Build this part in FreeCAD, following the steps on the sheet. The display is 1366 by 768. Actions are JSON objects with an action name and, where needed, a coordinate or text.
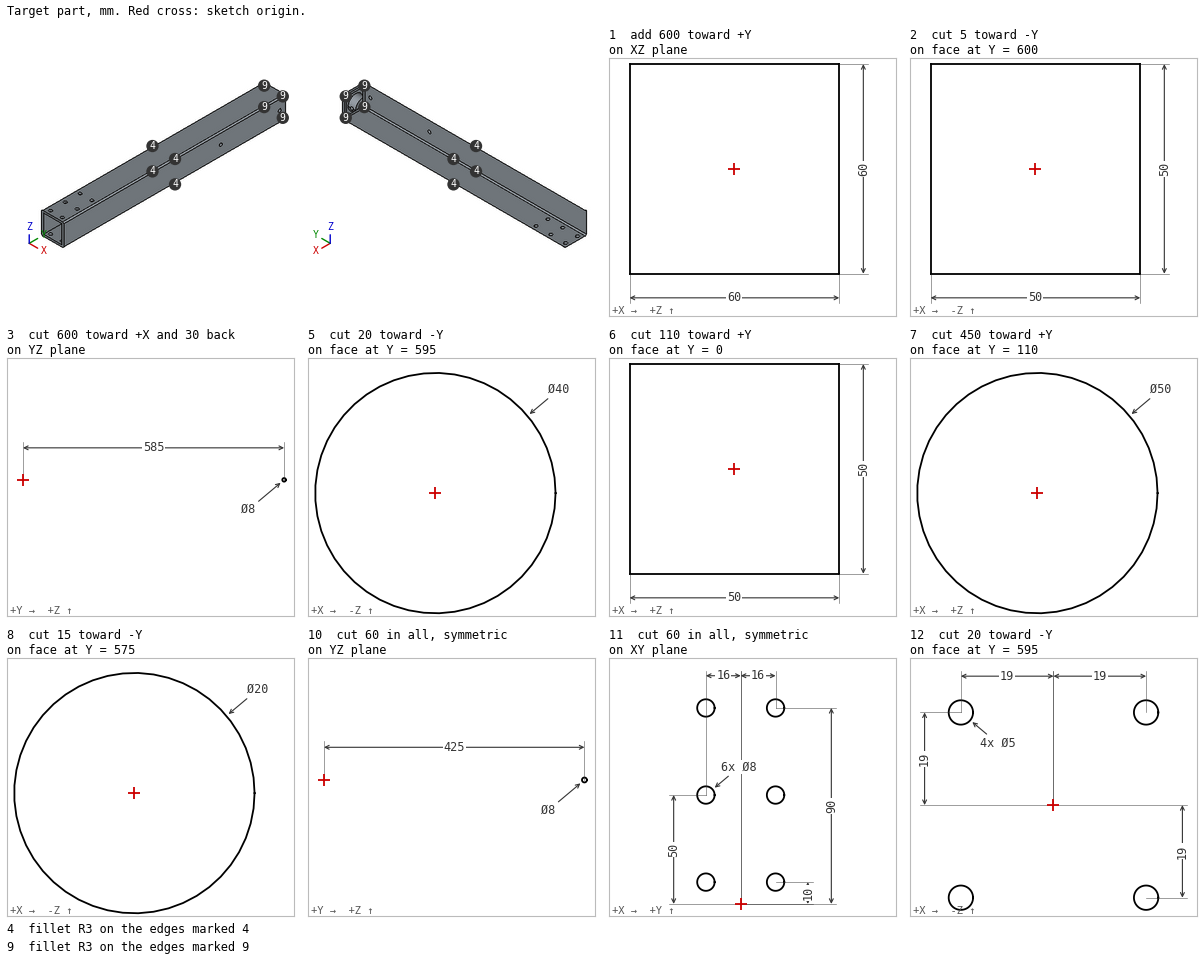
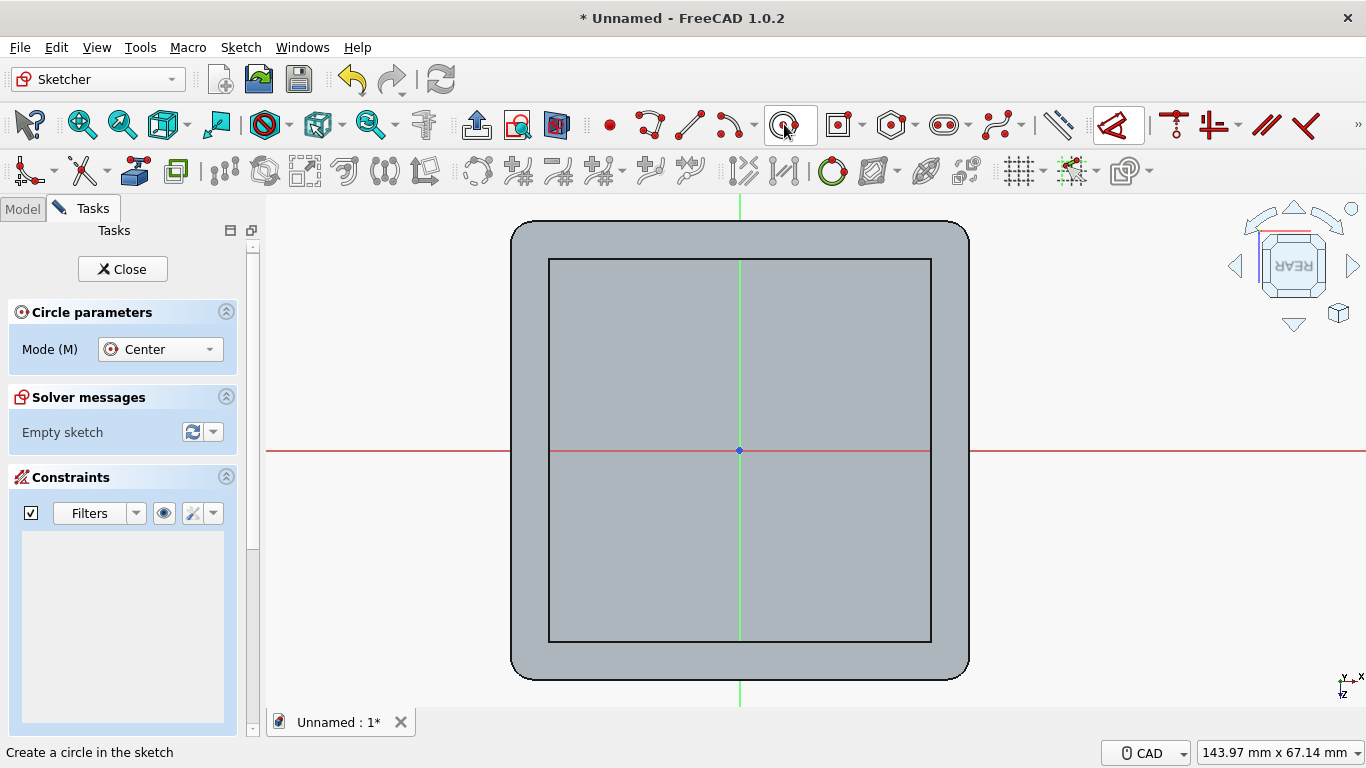
{"action": "left_click", "coordinate": [740, 450]}
{"action": "mouse_move", "coordinate": [848, 342]}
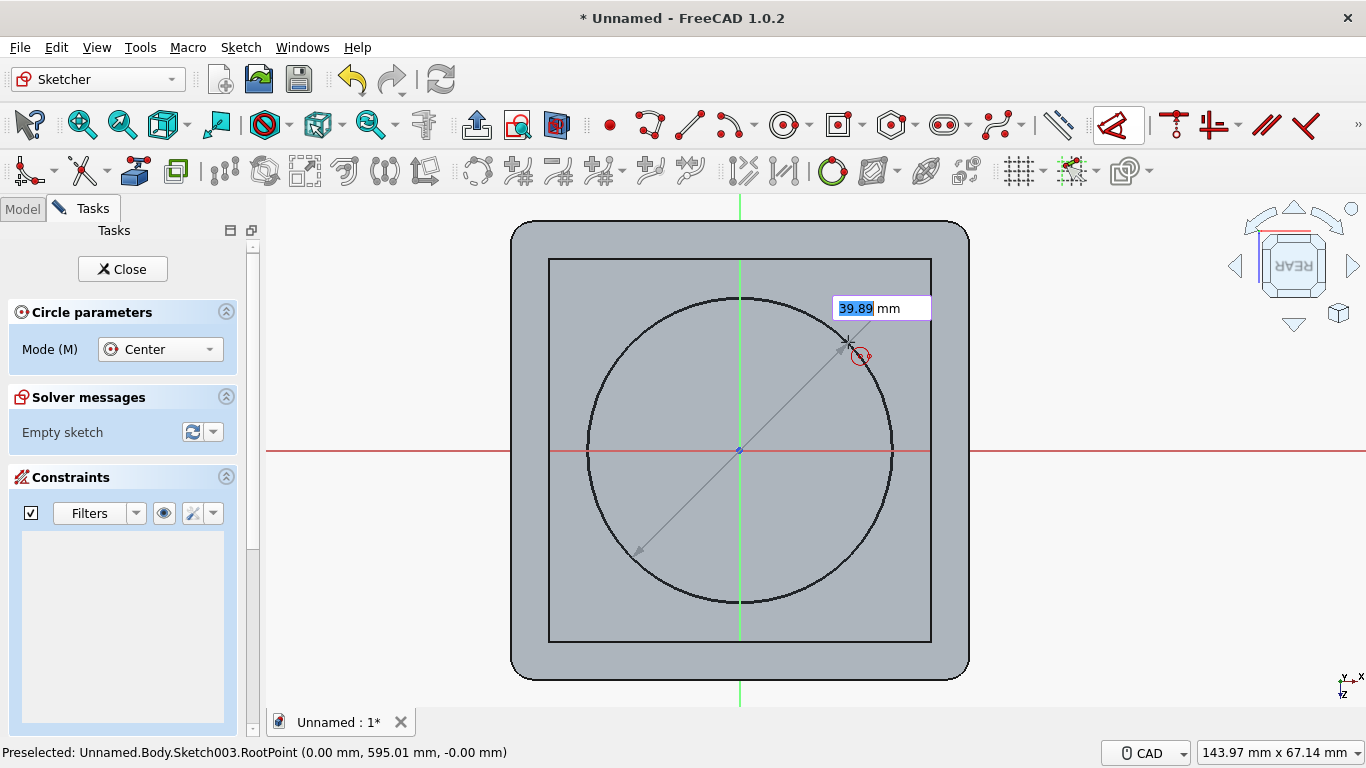
{"action": "type", "text": "40"}
{"action": "key", "text": "Return"}
{"action": "key", "text": "Escape"}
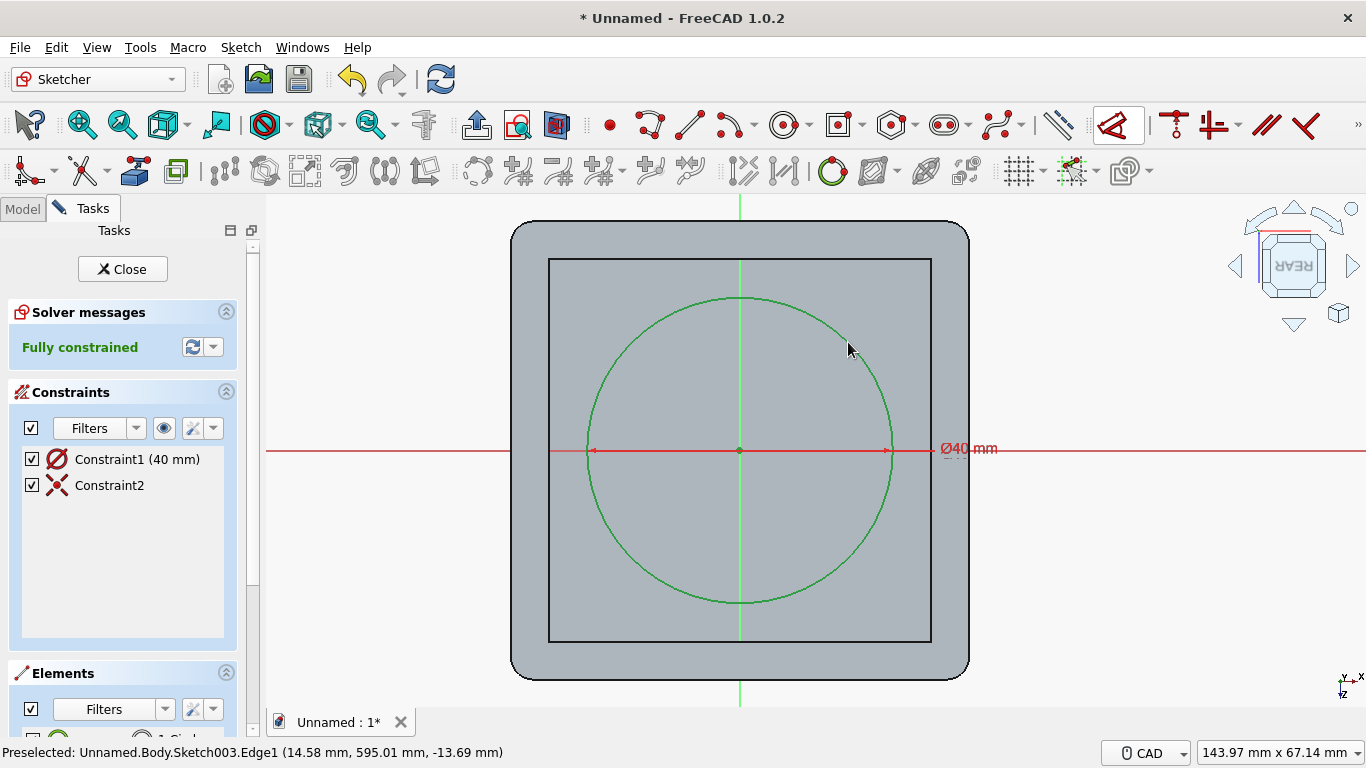
{"action": "left_click", "coordinate": [123, 269]}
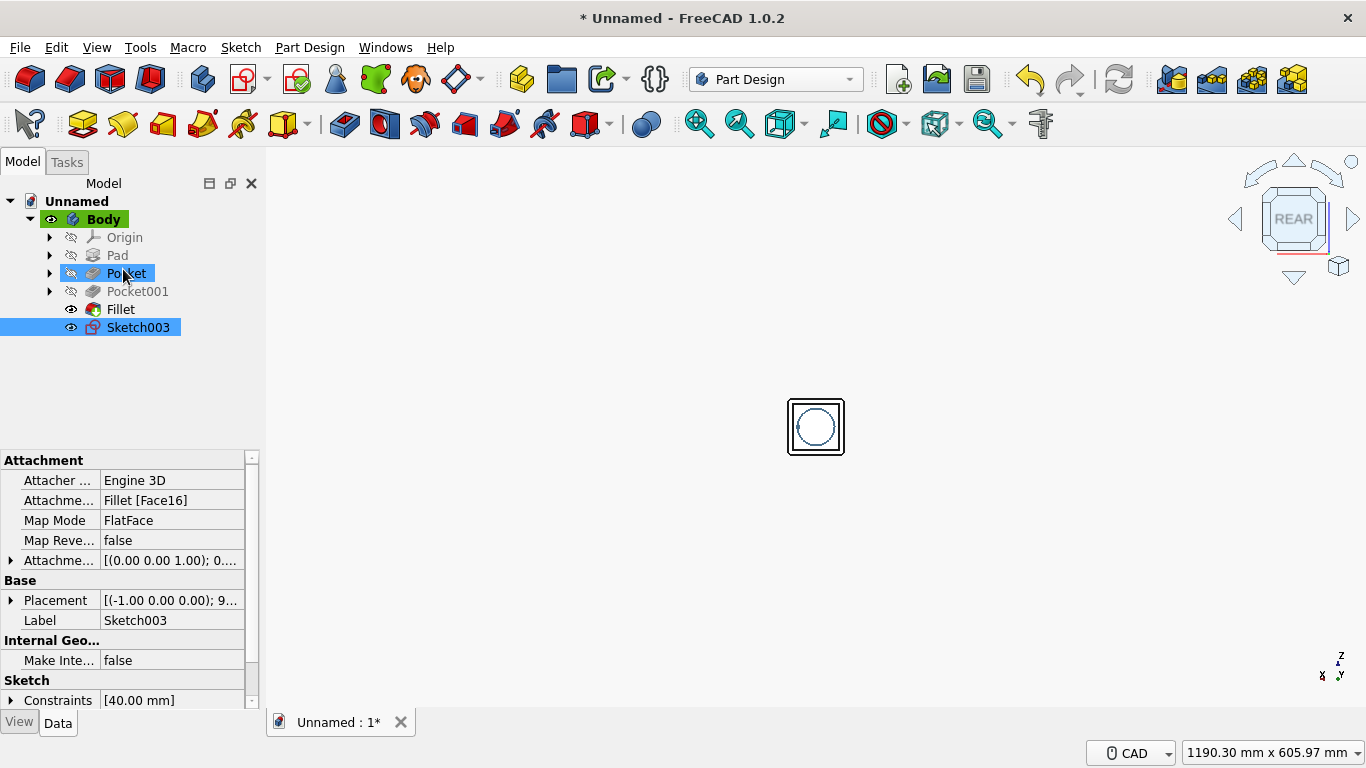
{"action": "left_click", "coordinate": [346, 124]}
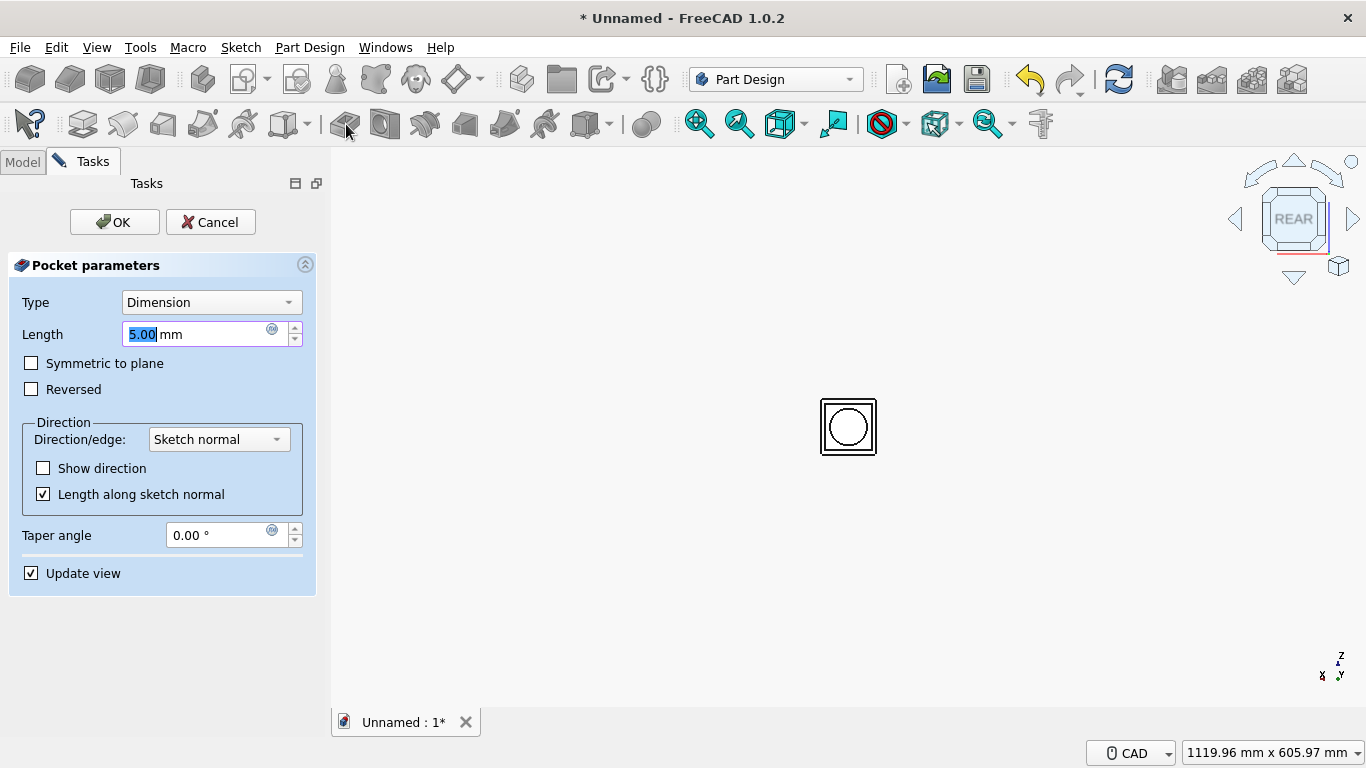
{"action": "type", "text": "20"}
{"action": "key", "text": "Tab"}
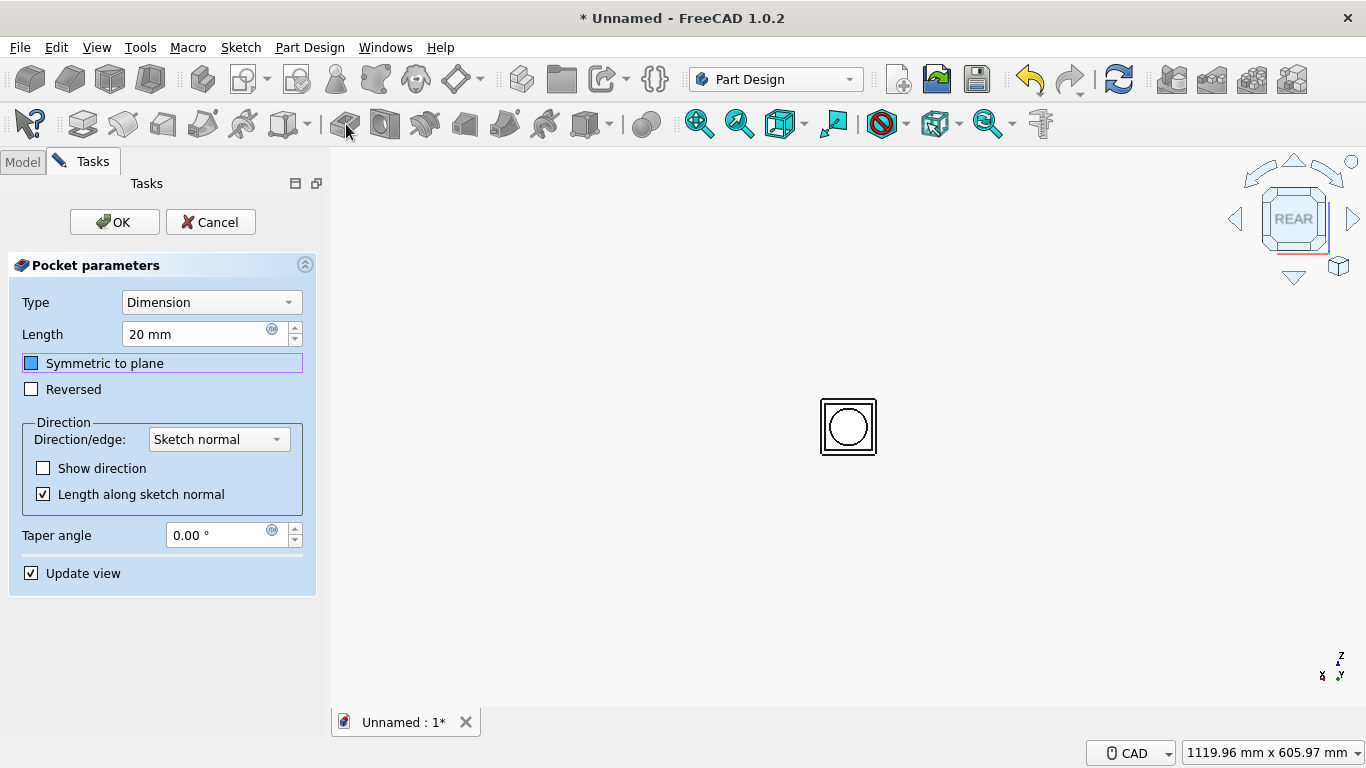
{"action": "left_click", "coordinate": [115, 222]}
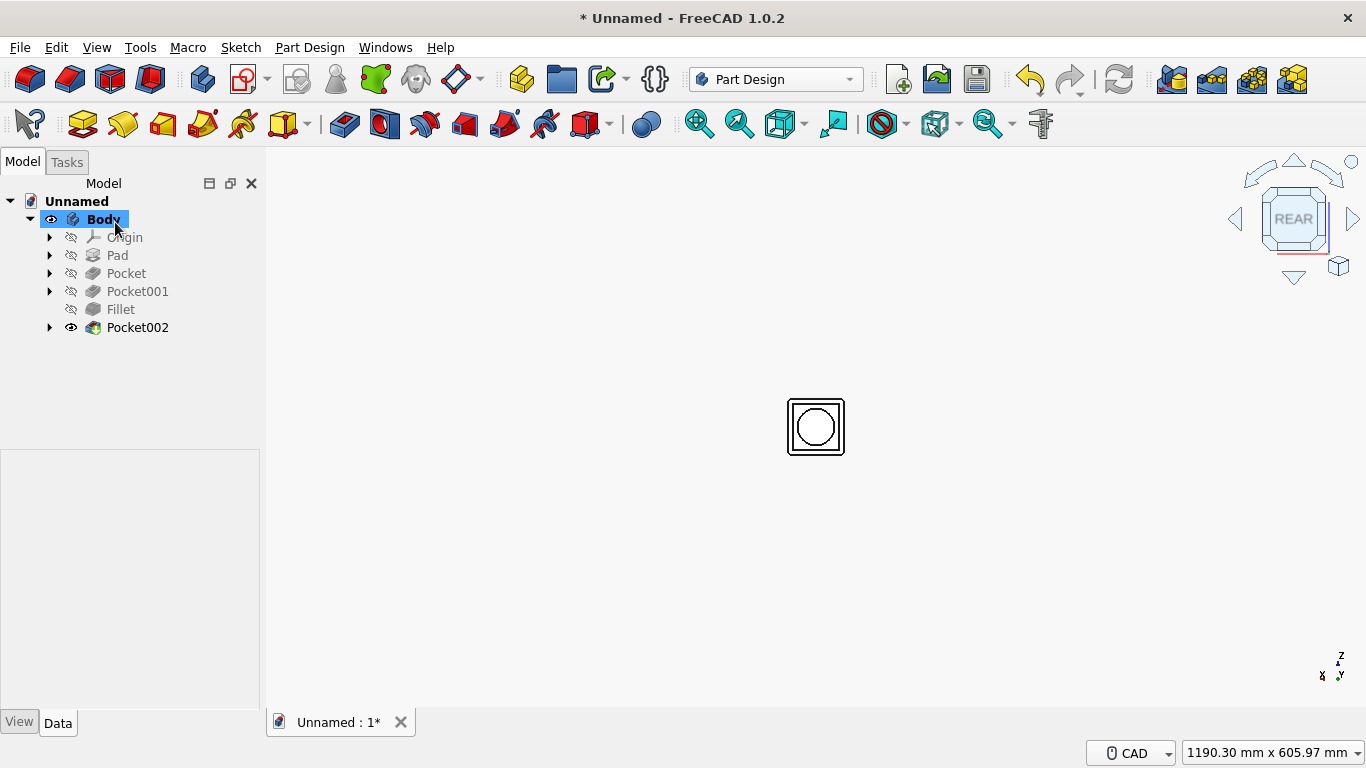
{"action": "left_click", "coordinate": [700, 124]}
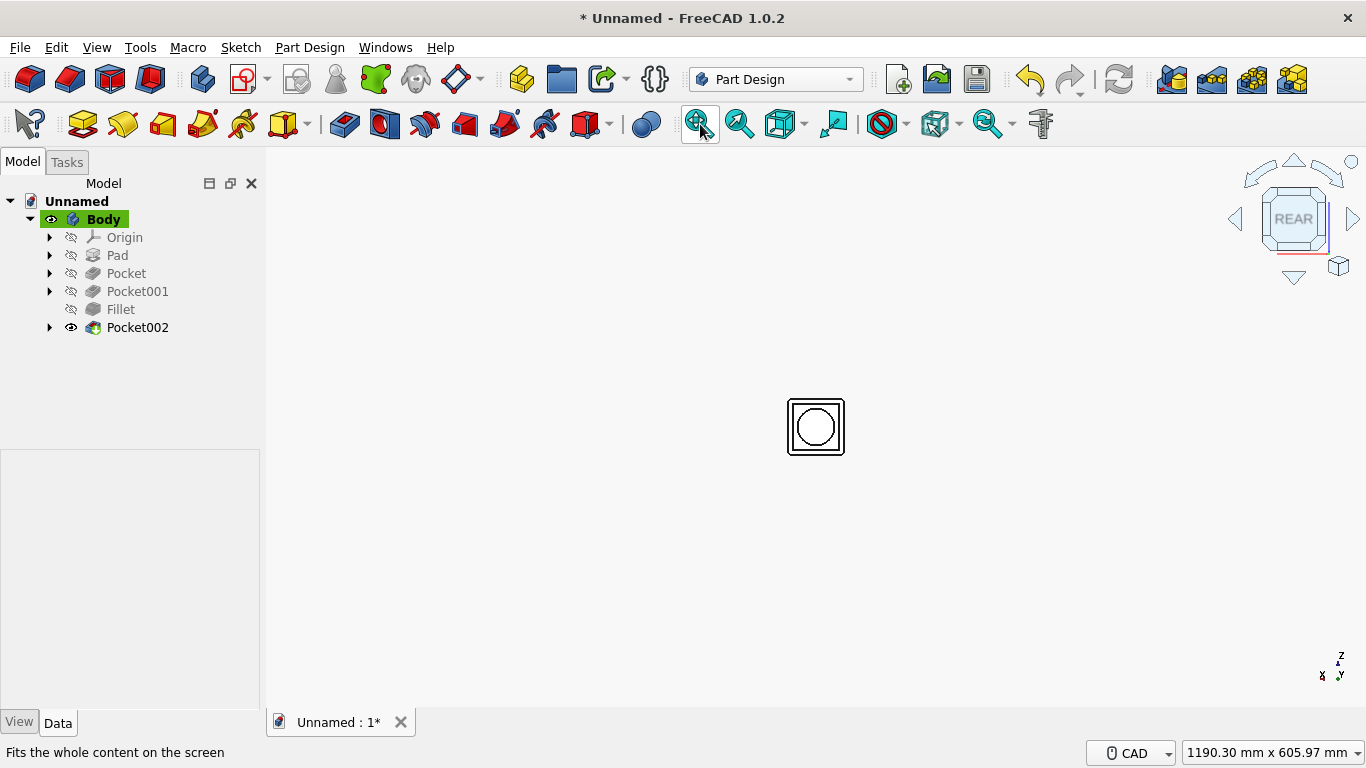
{"action": "key", "text": "0"}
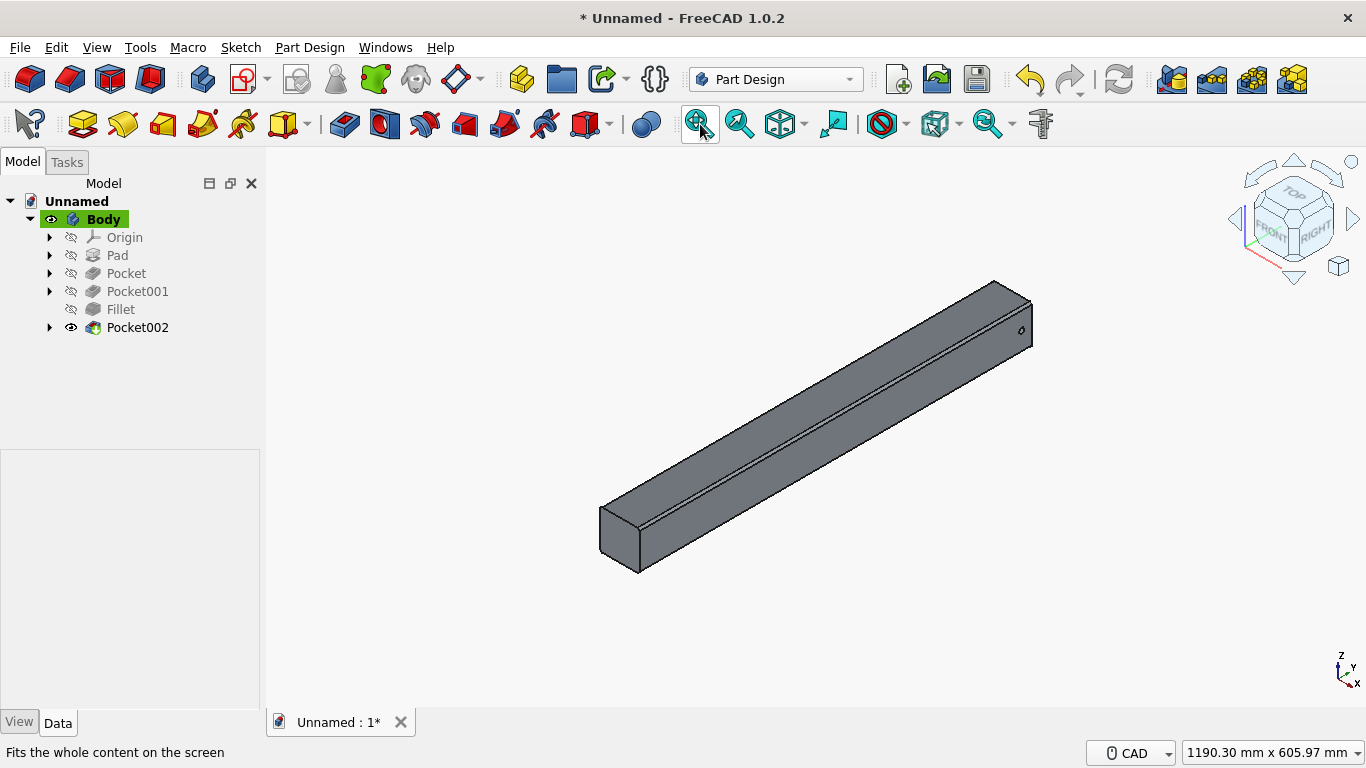
{"action": "left_click", "coordinate": [620, 539]}